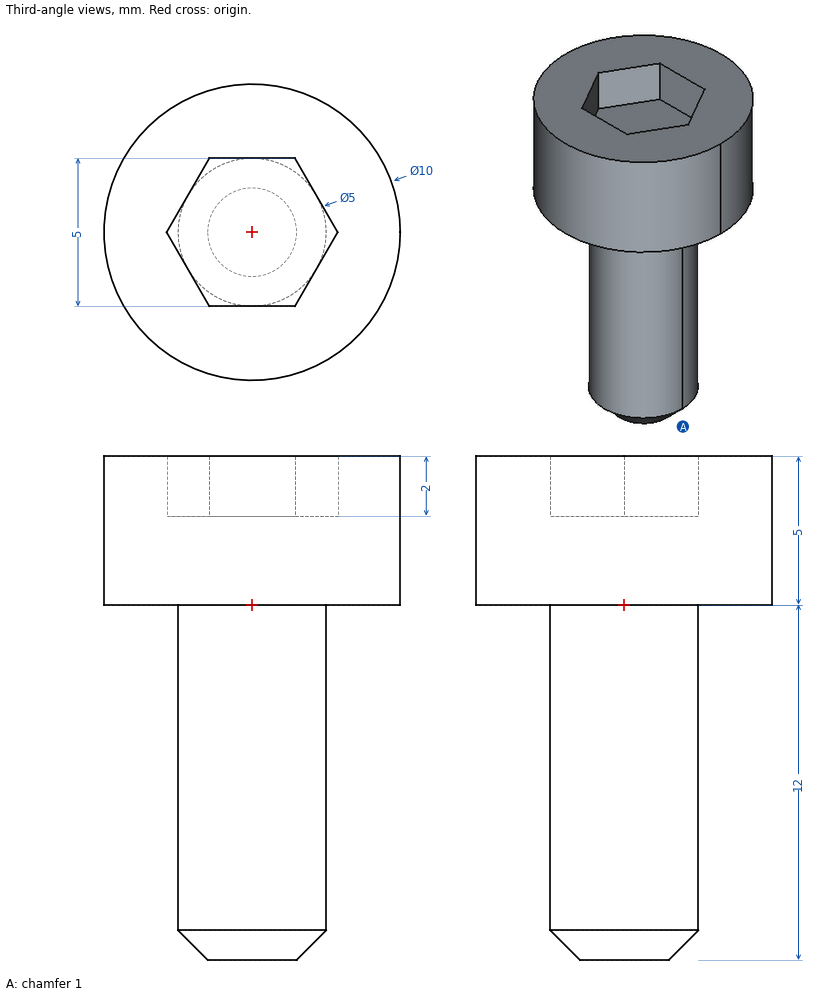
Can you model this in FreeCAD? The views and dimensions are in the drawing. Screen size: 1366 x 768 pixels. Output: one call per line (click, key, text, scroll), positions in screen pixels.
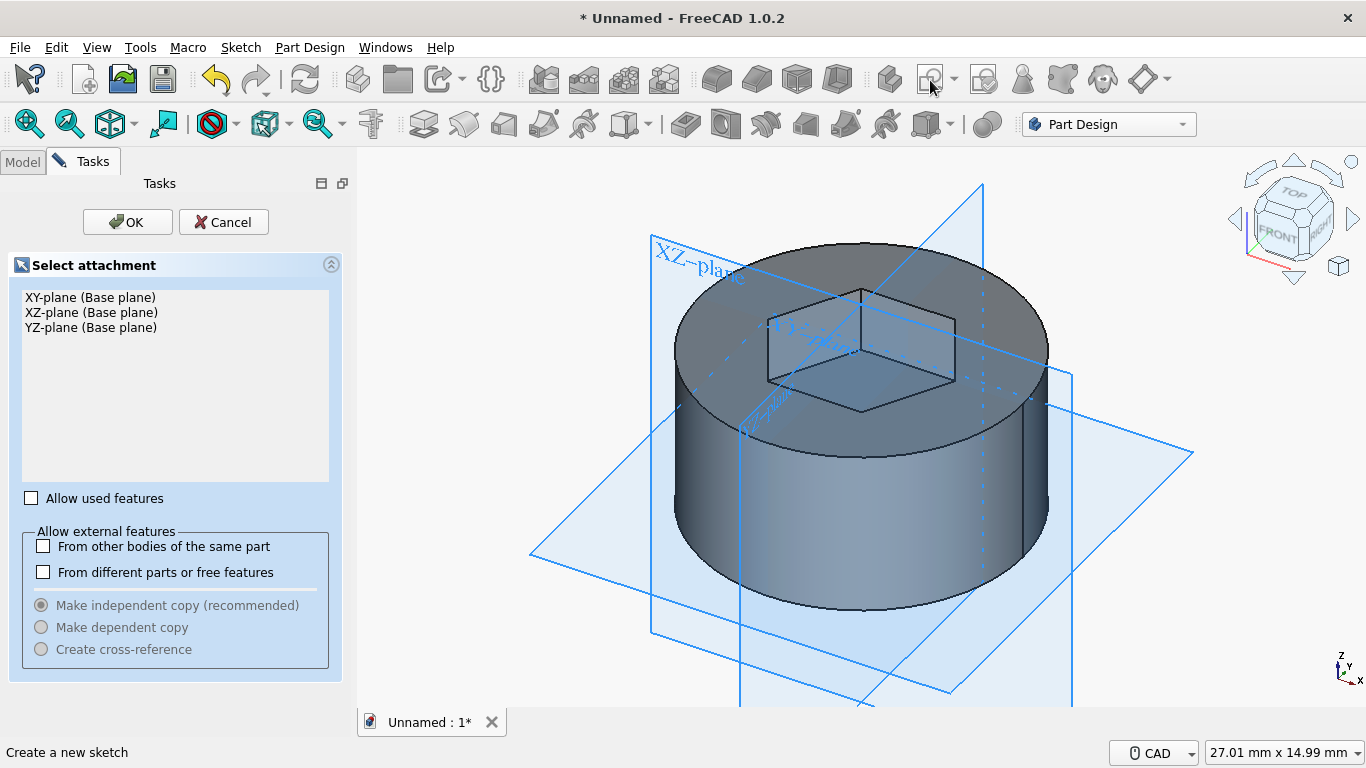
click(82, 298)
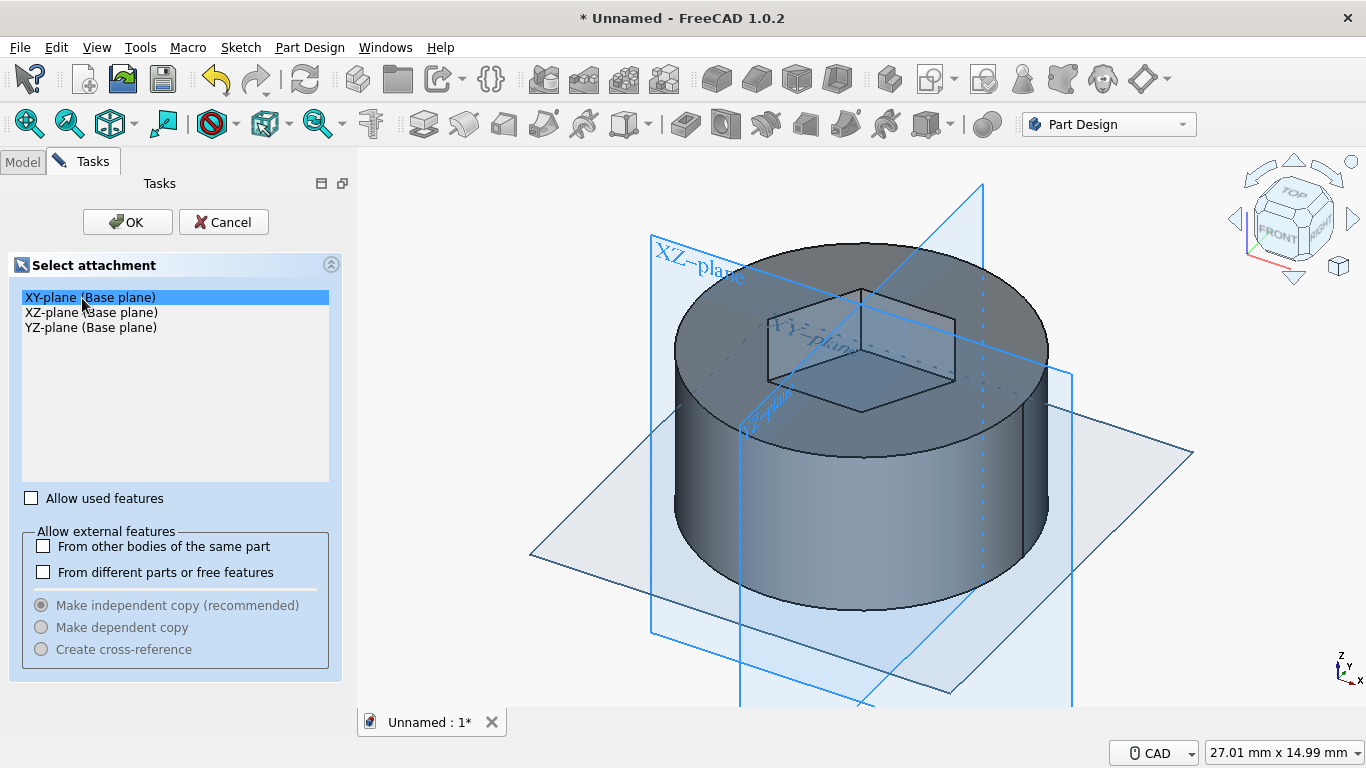
click(128, 222)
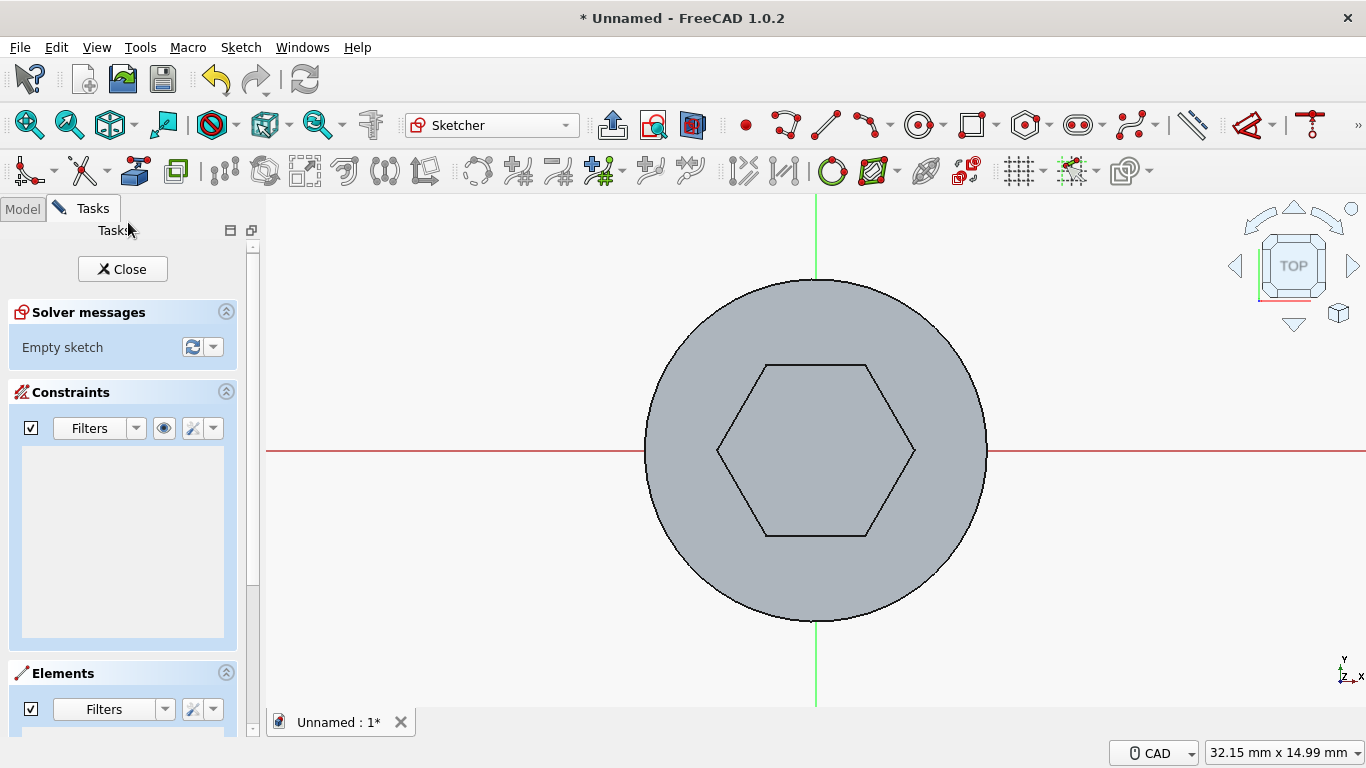
key(q)
key(s)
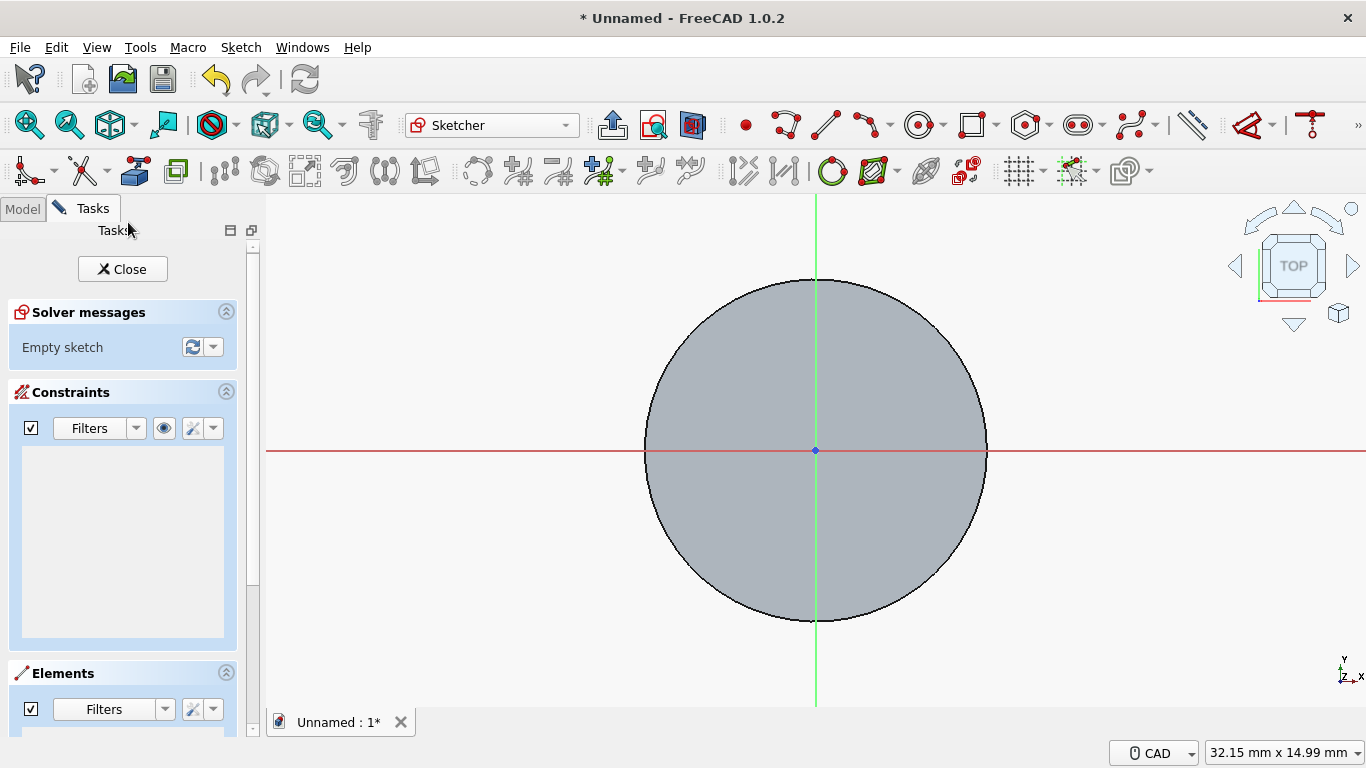
scroll(899, 450, up, 3)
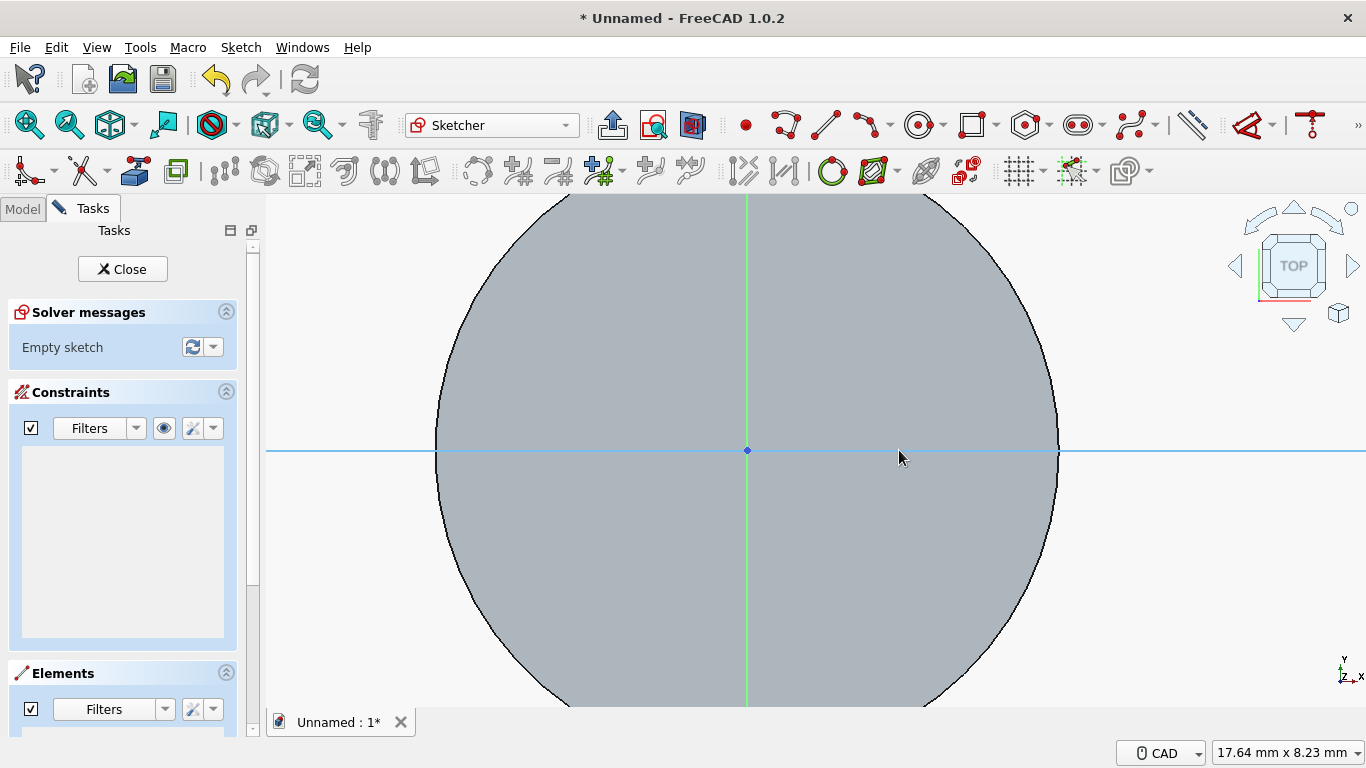
key(g)
key(c)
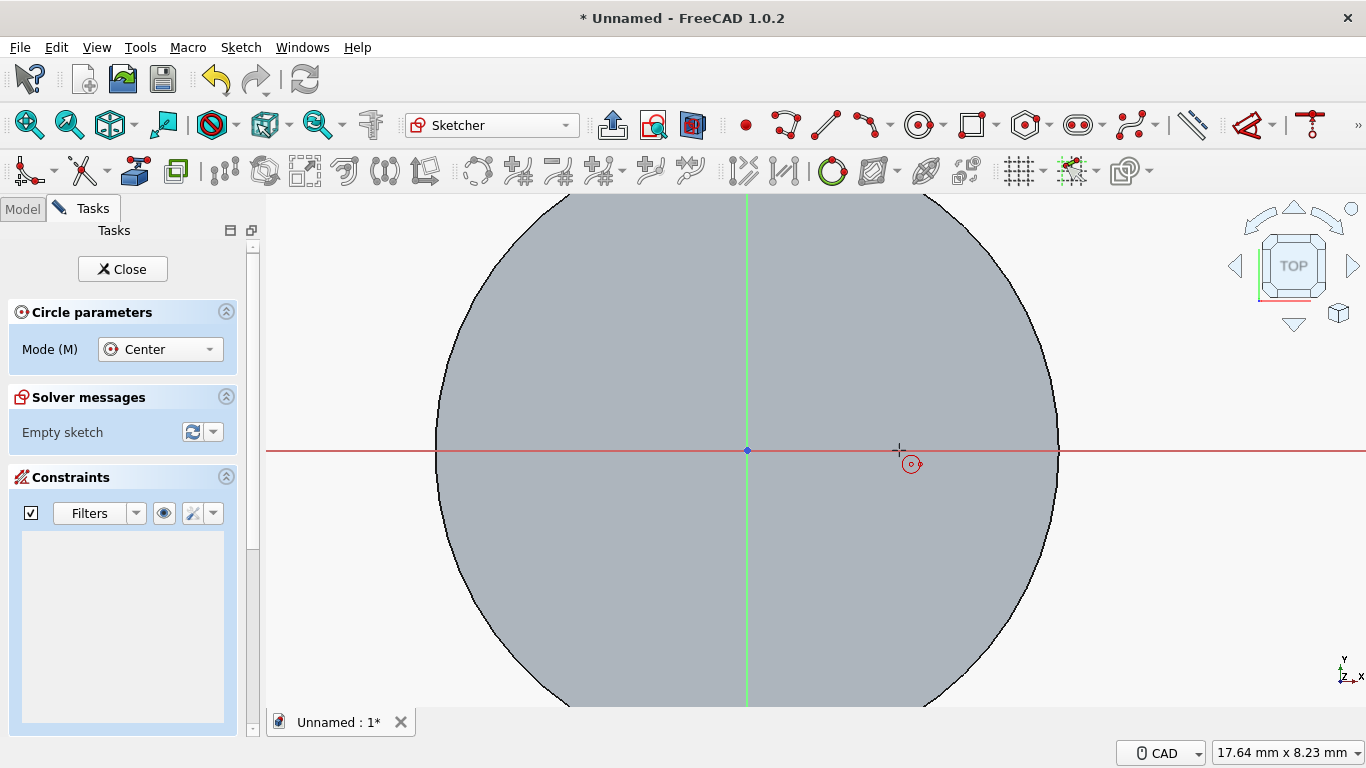
click(747, 450)
click(857, 340)
key(Escape)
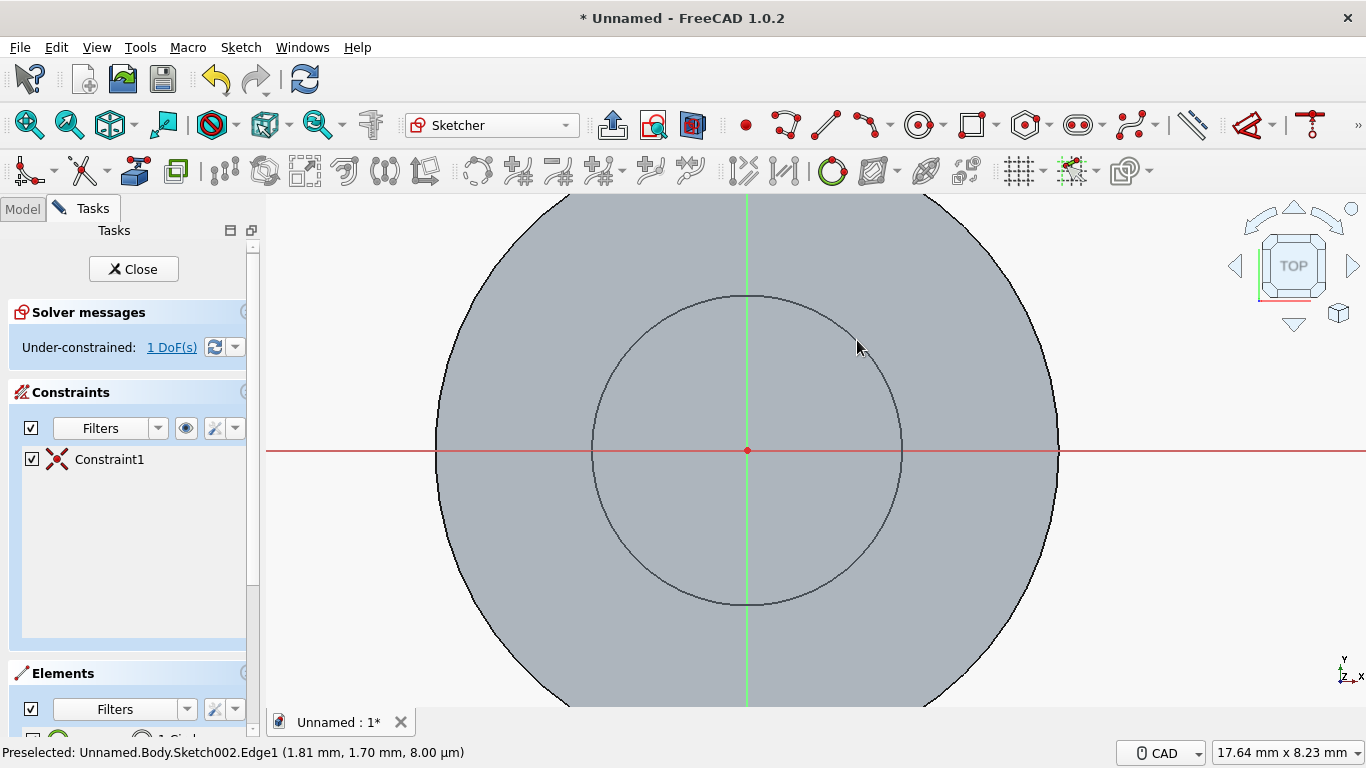
key(d)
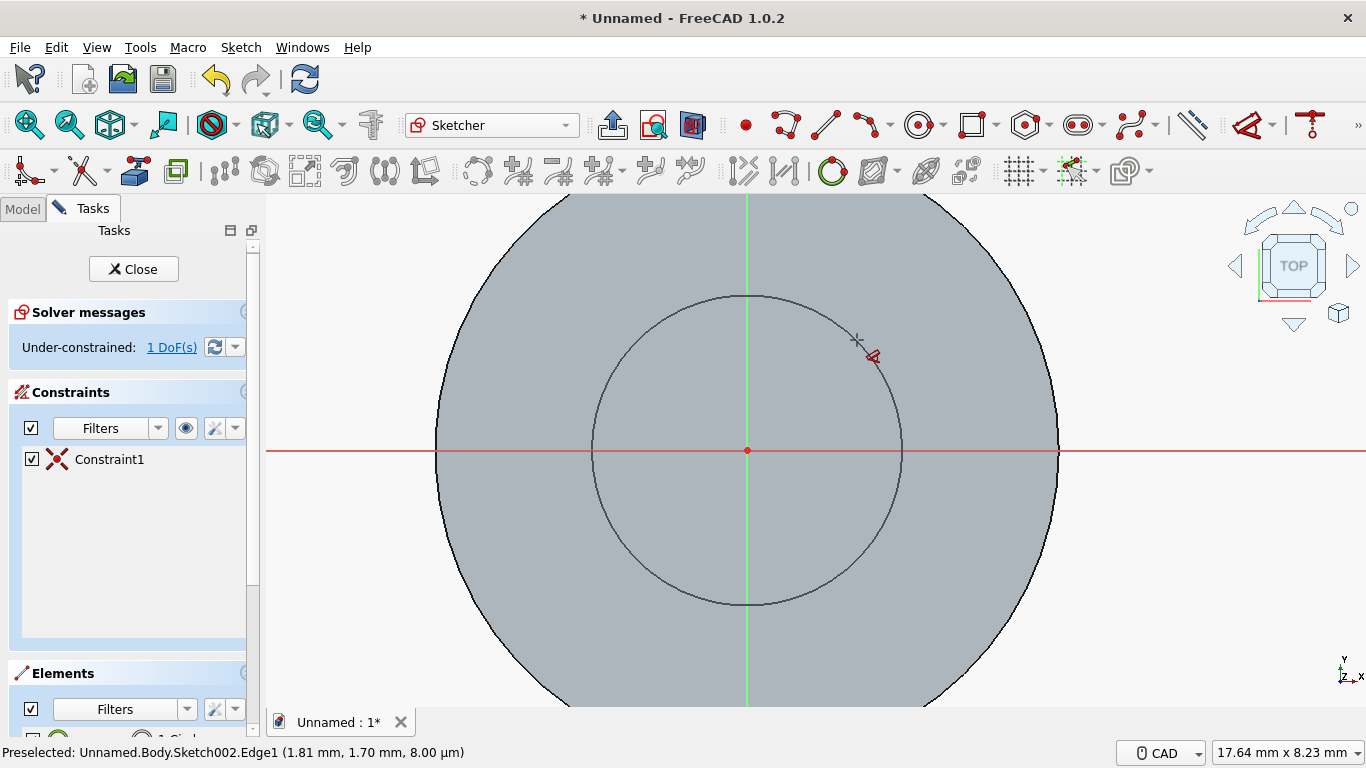
click(856, 340)
click(878, 317)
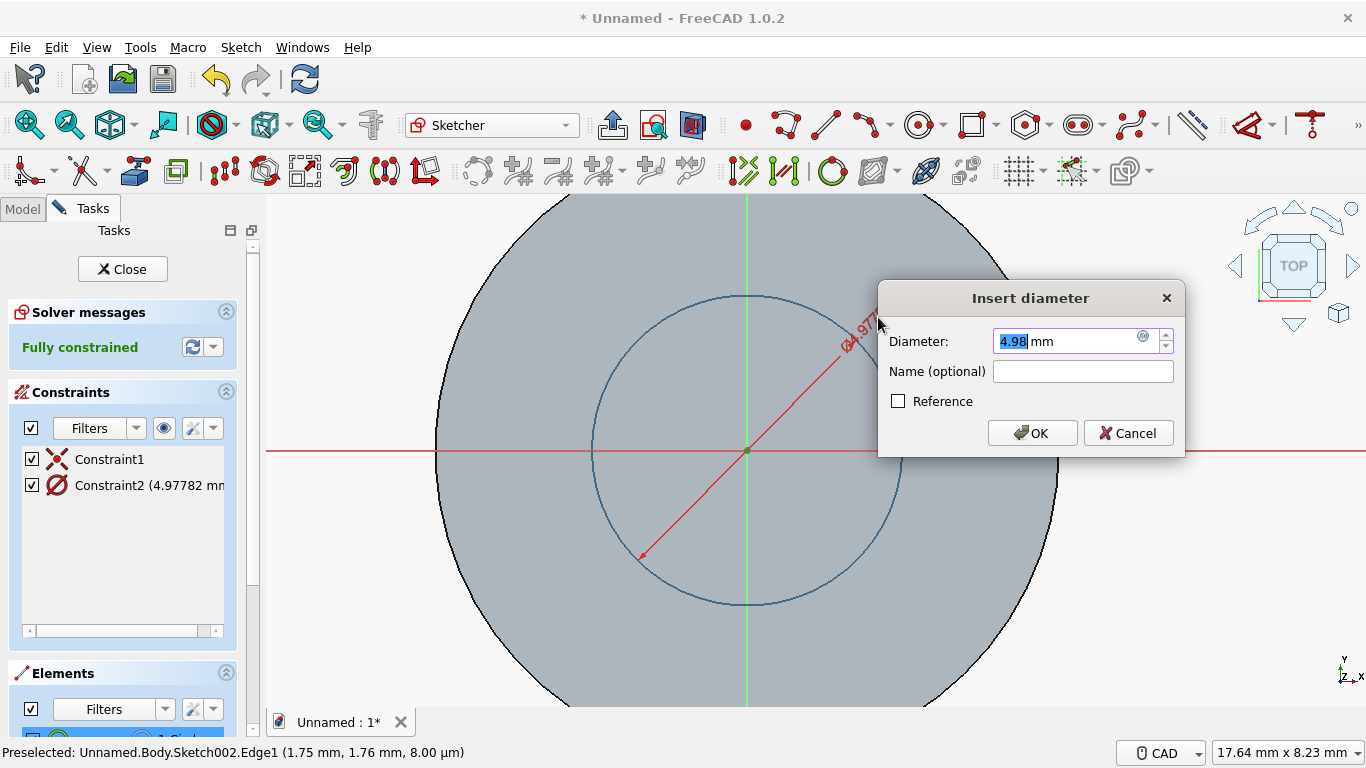
text(5)
key(Return)
key(Escape)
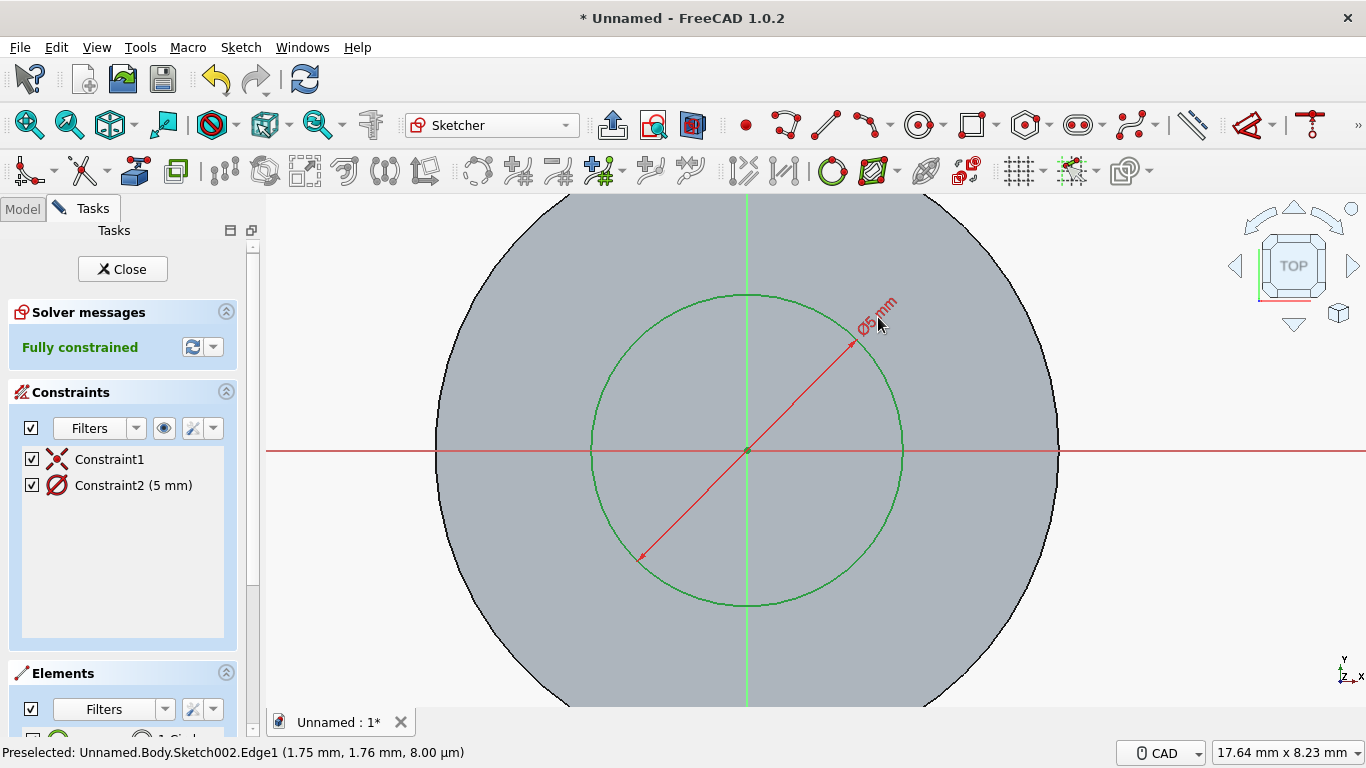
click(123, 269)